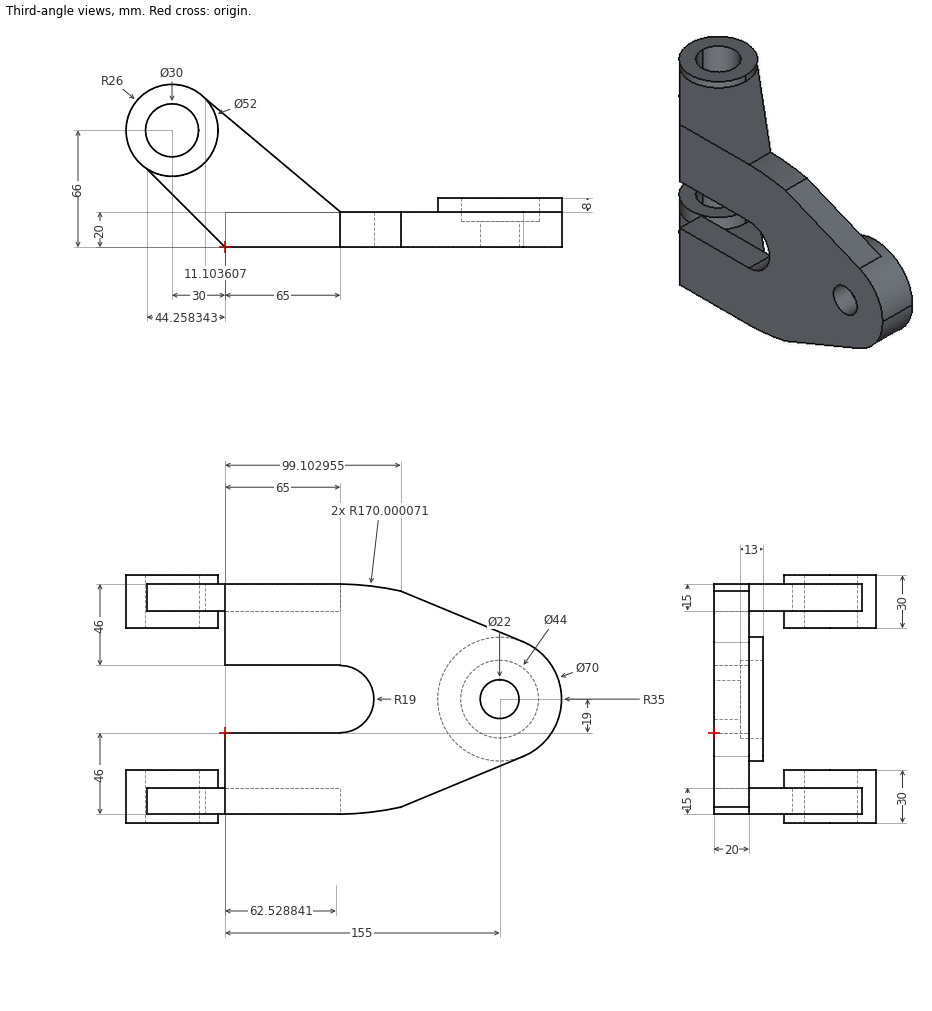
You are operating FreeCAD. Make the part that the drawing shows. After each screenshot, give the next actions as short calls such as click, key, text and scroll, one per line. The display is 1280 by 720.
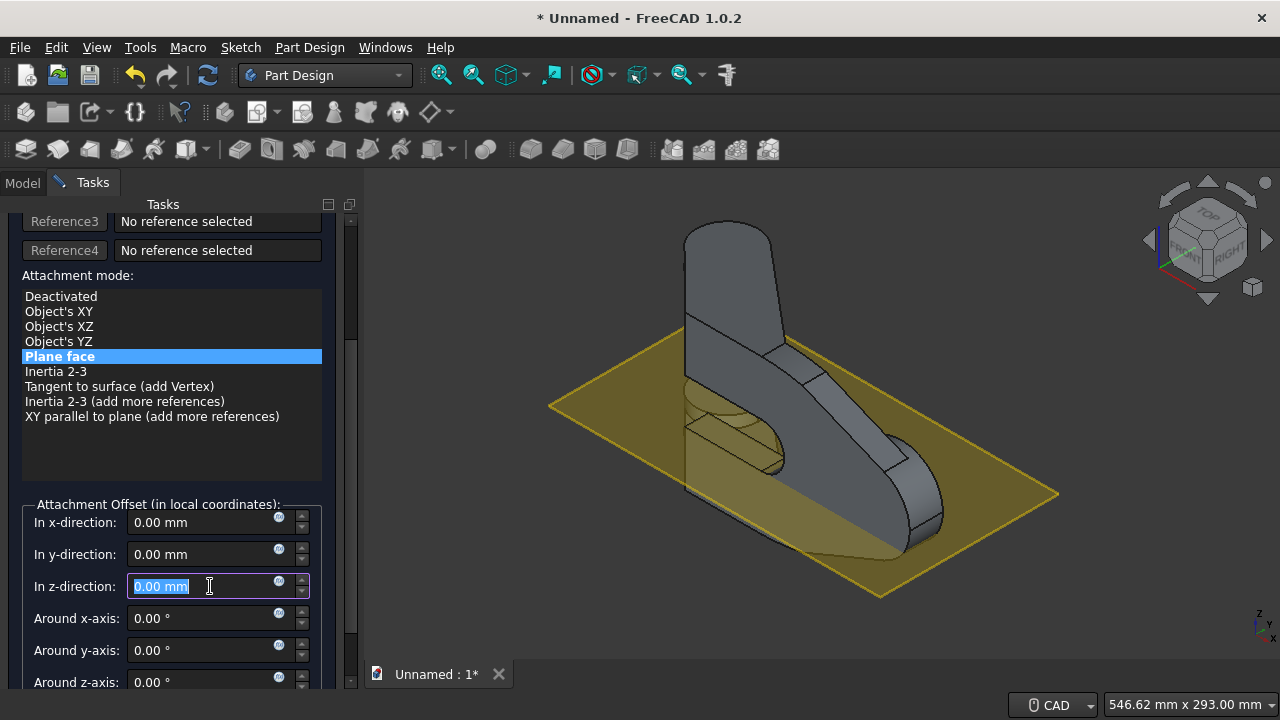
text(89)
key(Tab)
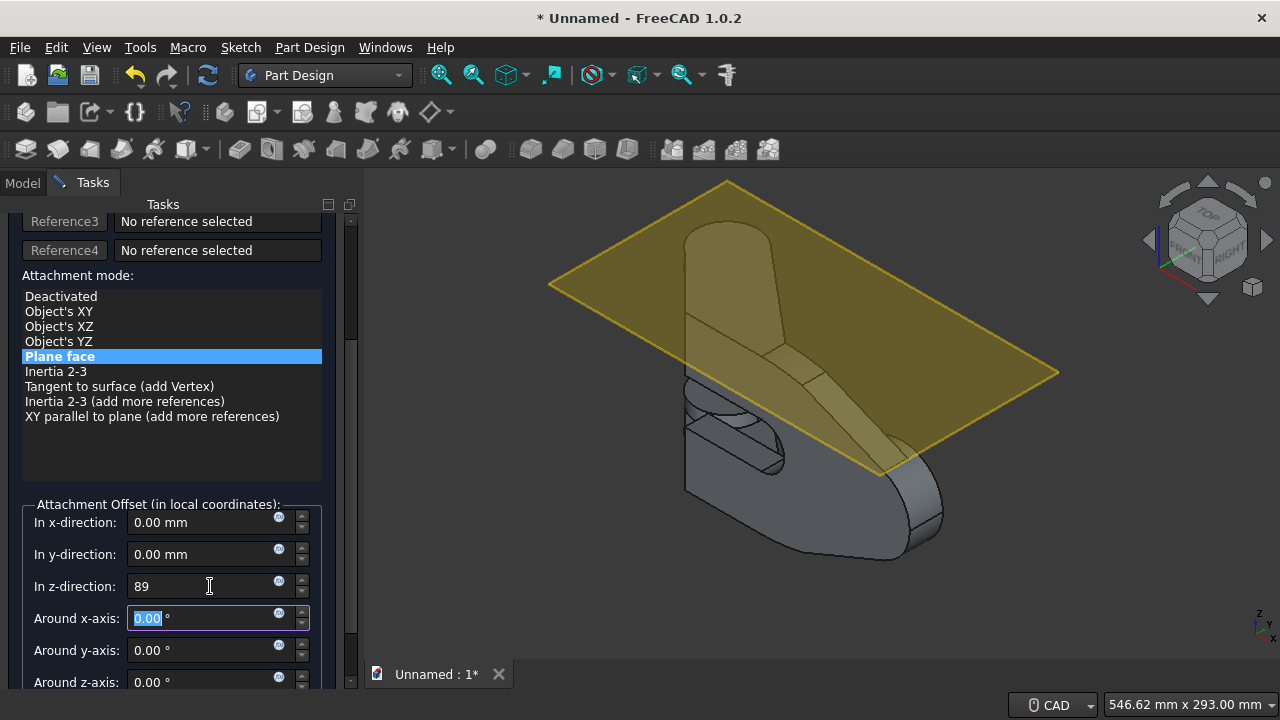
scroll(351, 451, up, 4)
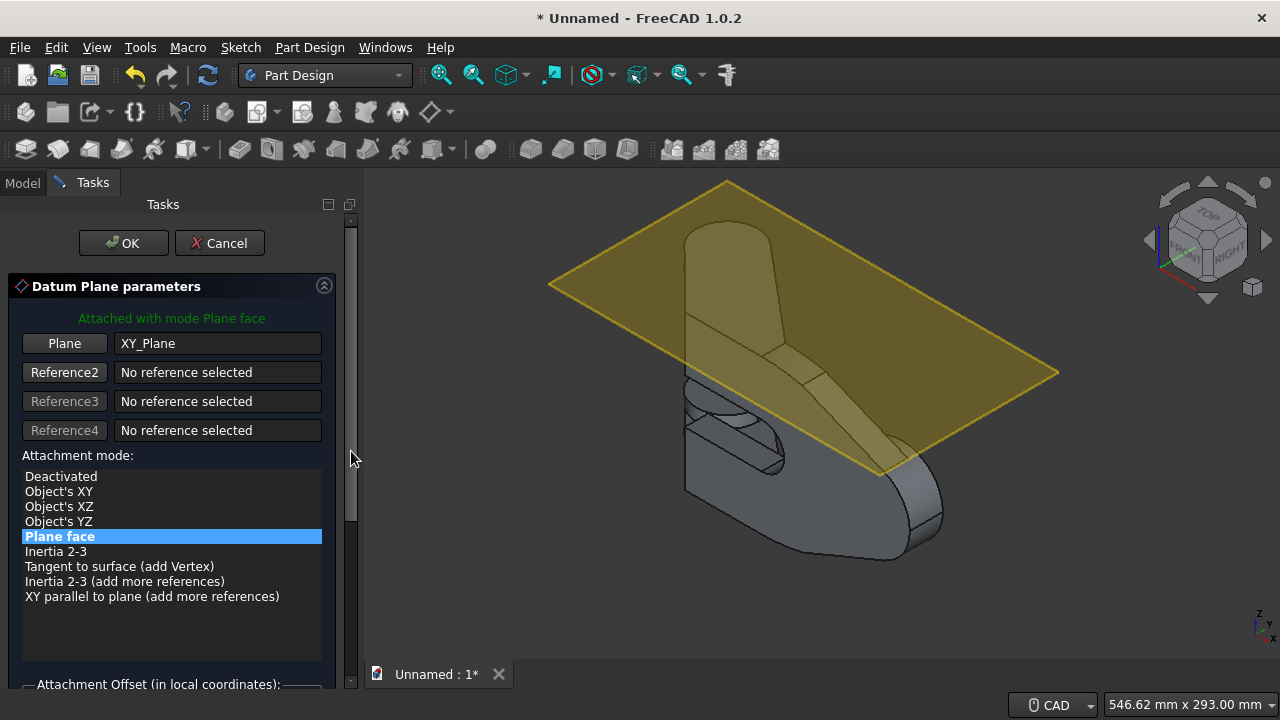
click(124, 243)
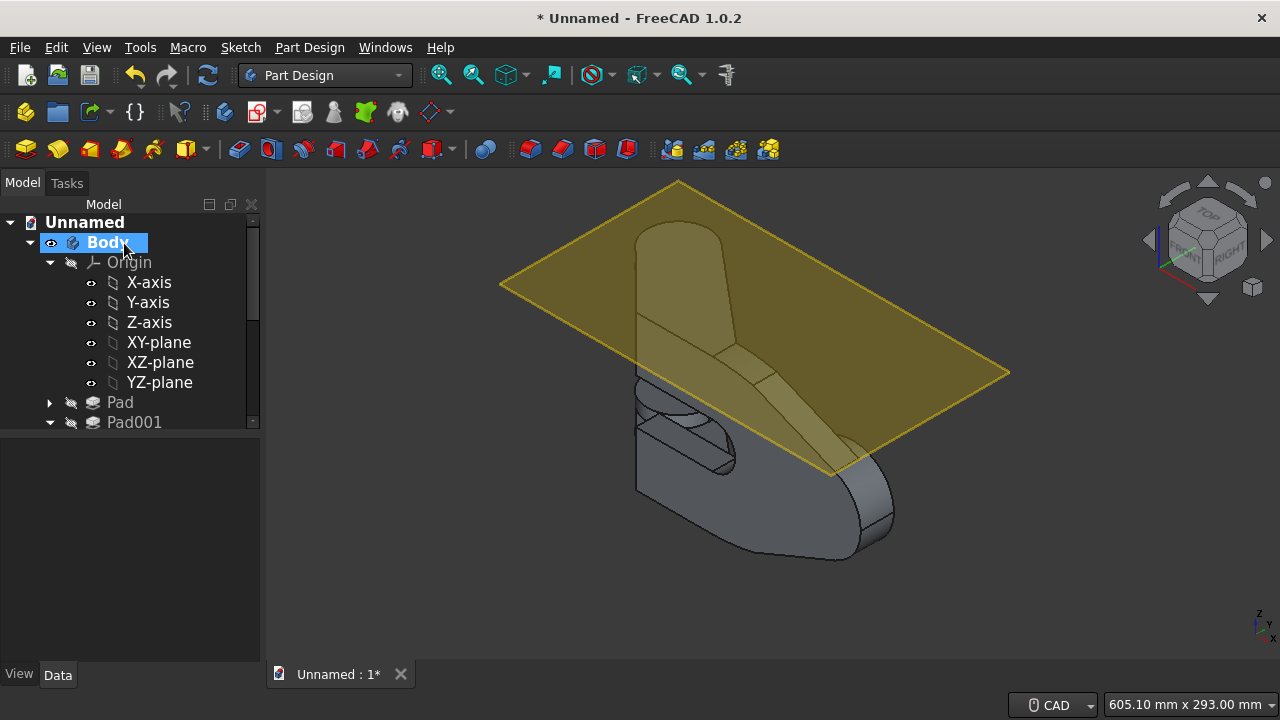
scroll(100, 318, down, 3)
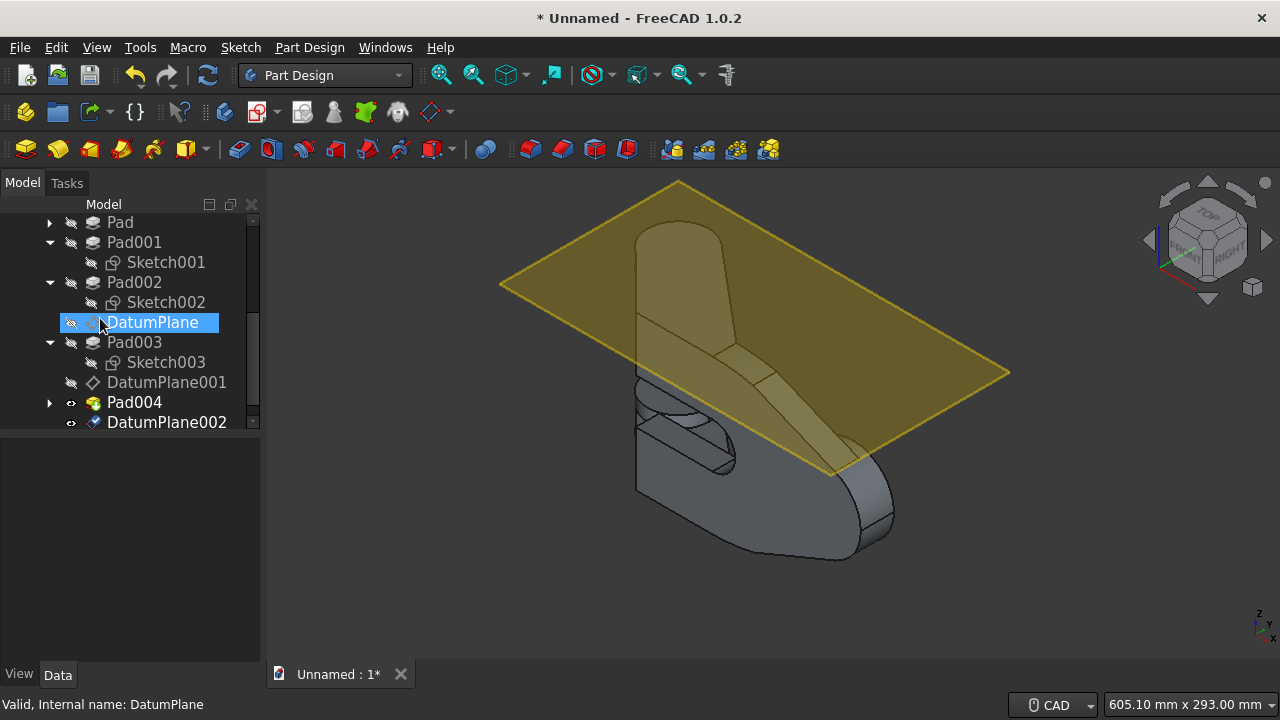
click(116, 423)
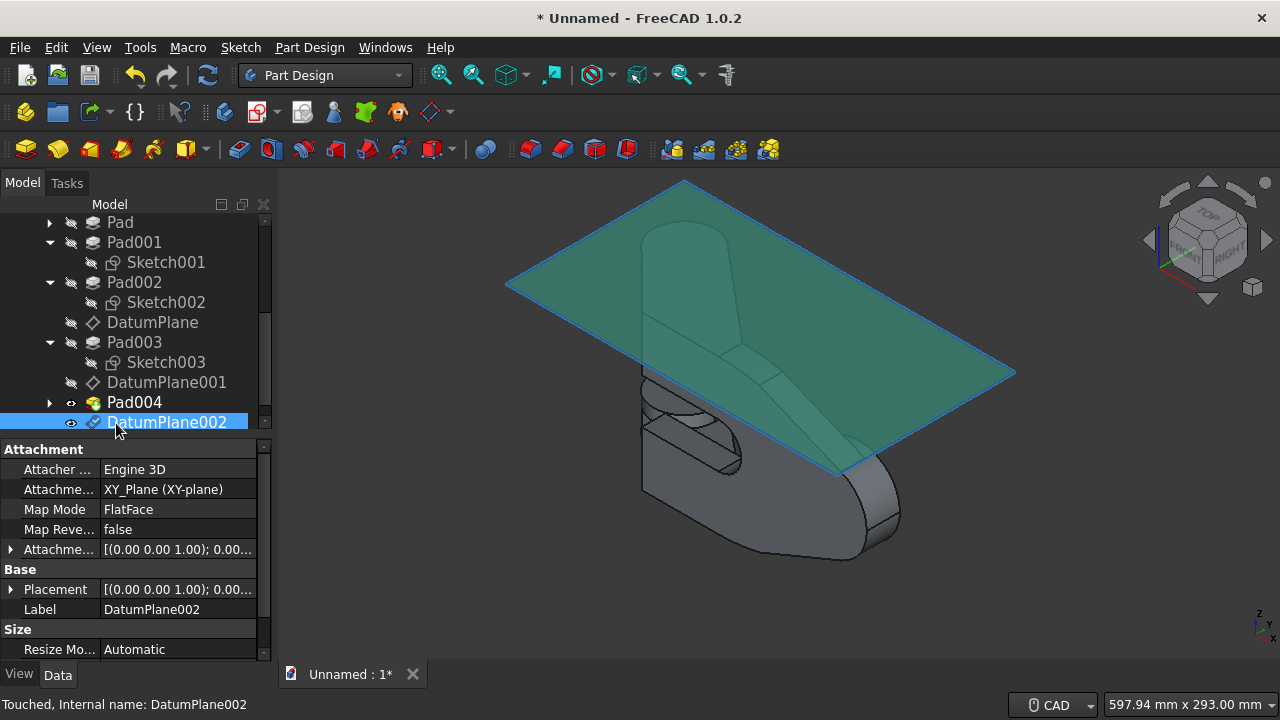
click(258, 112)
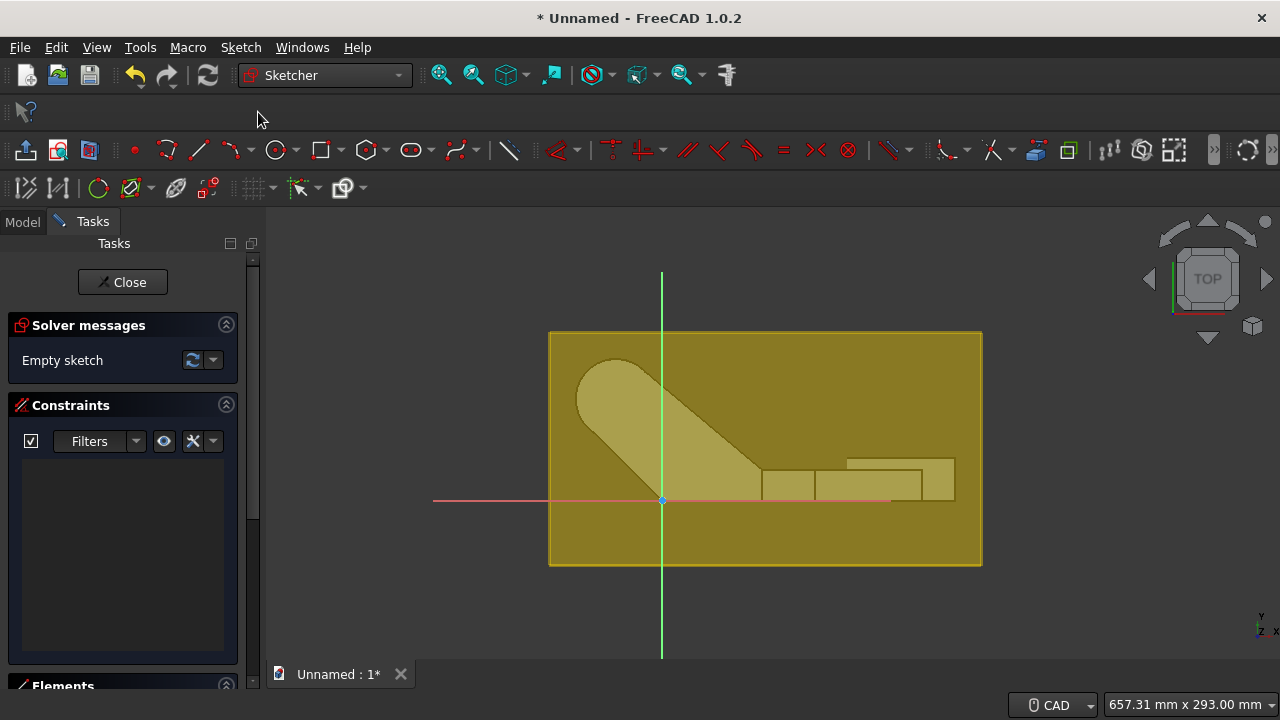
scroll(515, 426, up, 3)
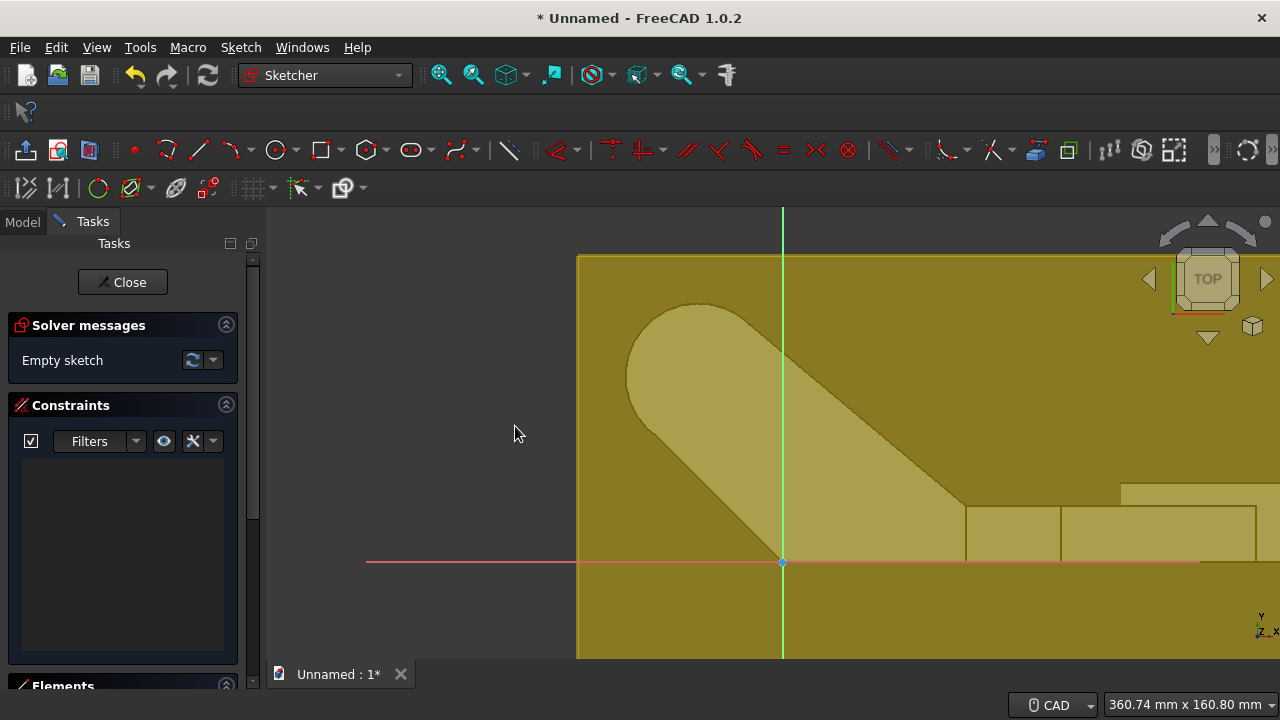
key(g)
key(c)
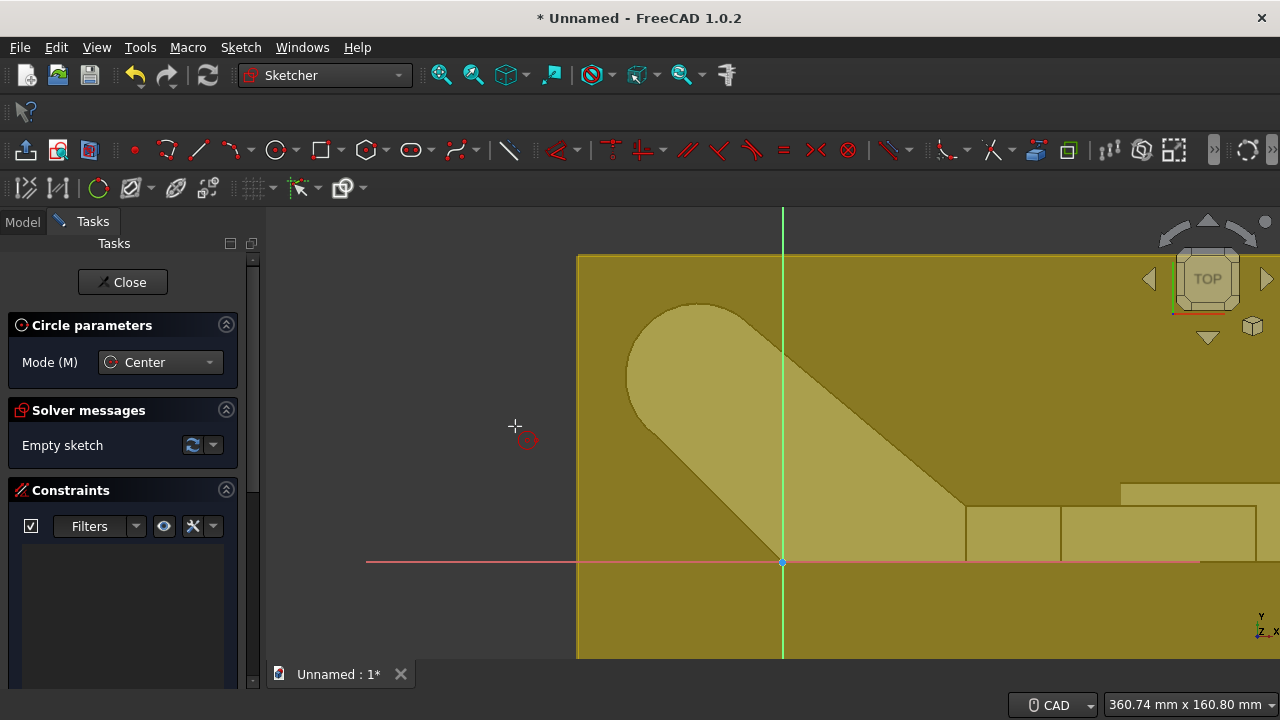
click(699, 377)
move(750, 325)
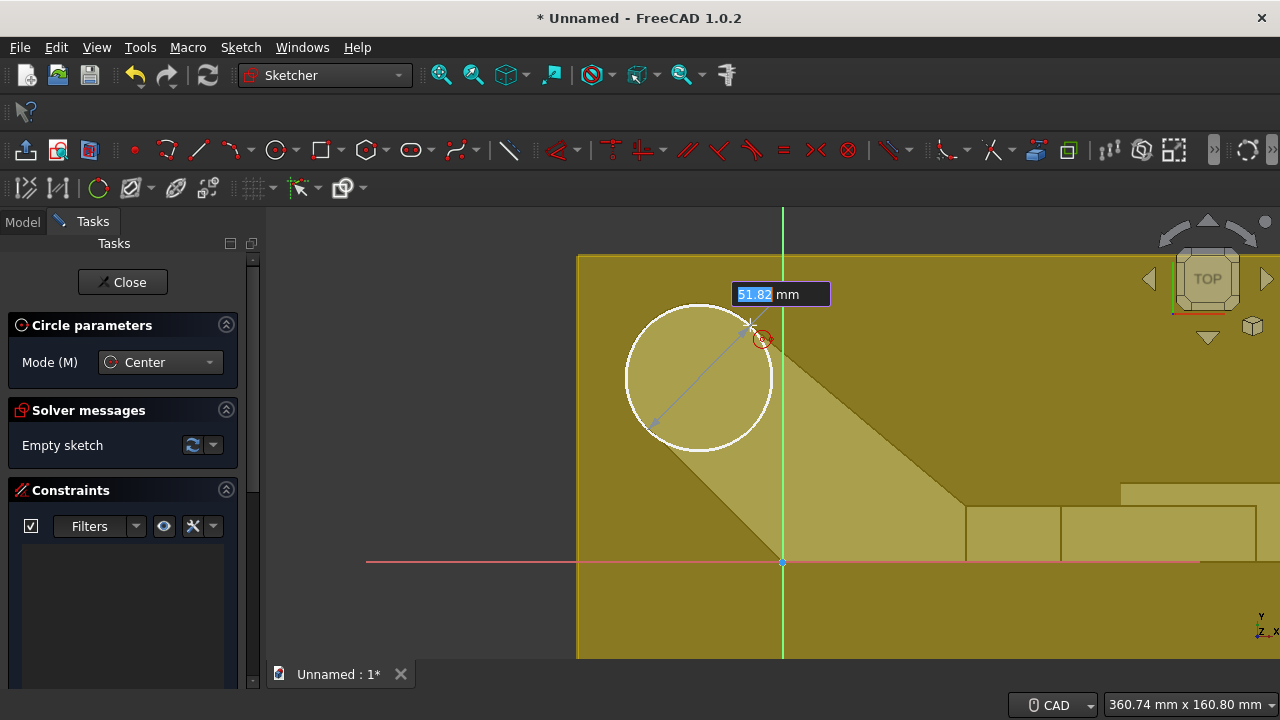
text(52)
key(Return)
key(Escape)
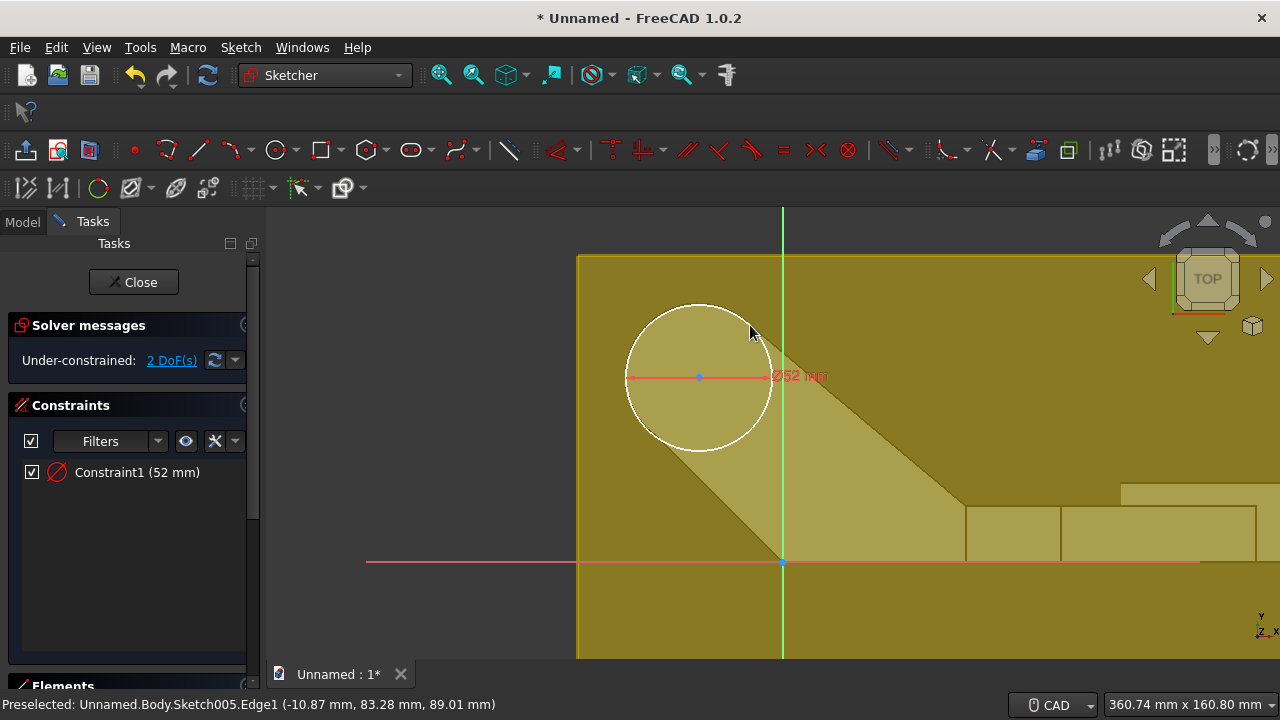
click(556, 150)